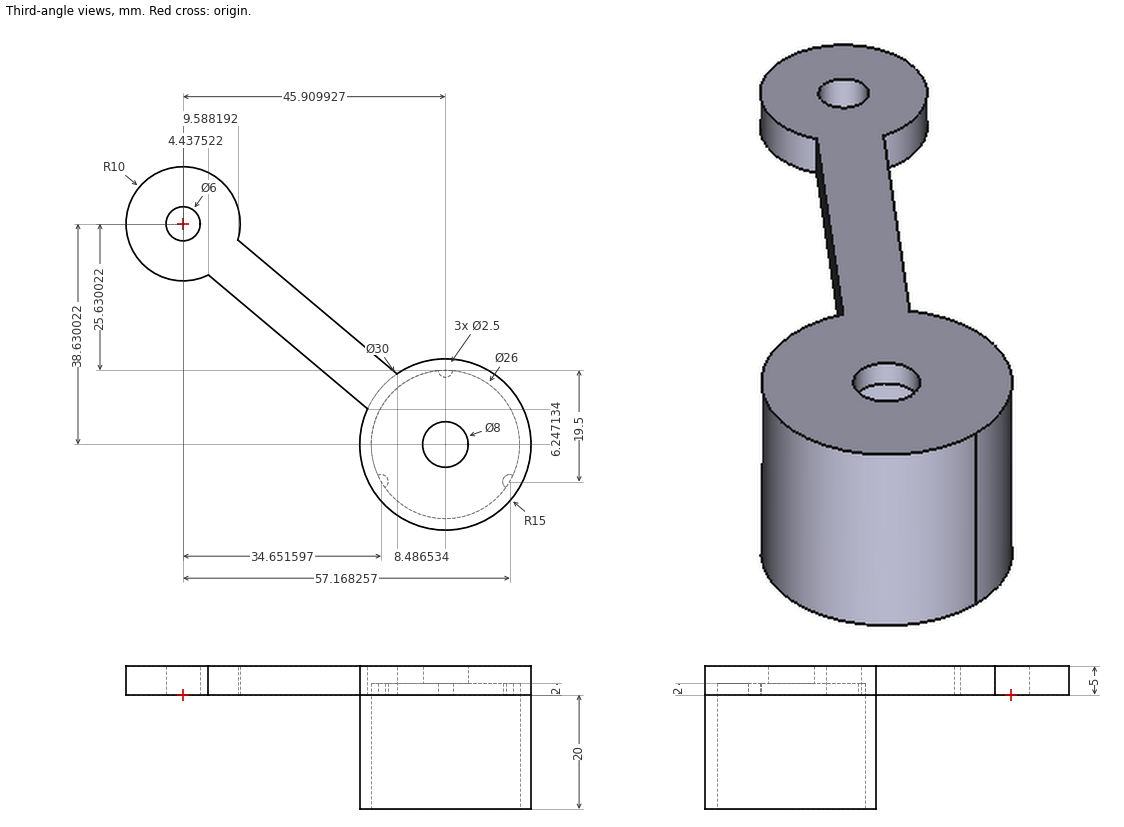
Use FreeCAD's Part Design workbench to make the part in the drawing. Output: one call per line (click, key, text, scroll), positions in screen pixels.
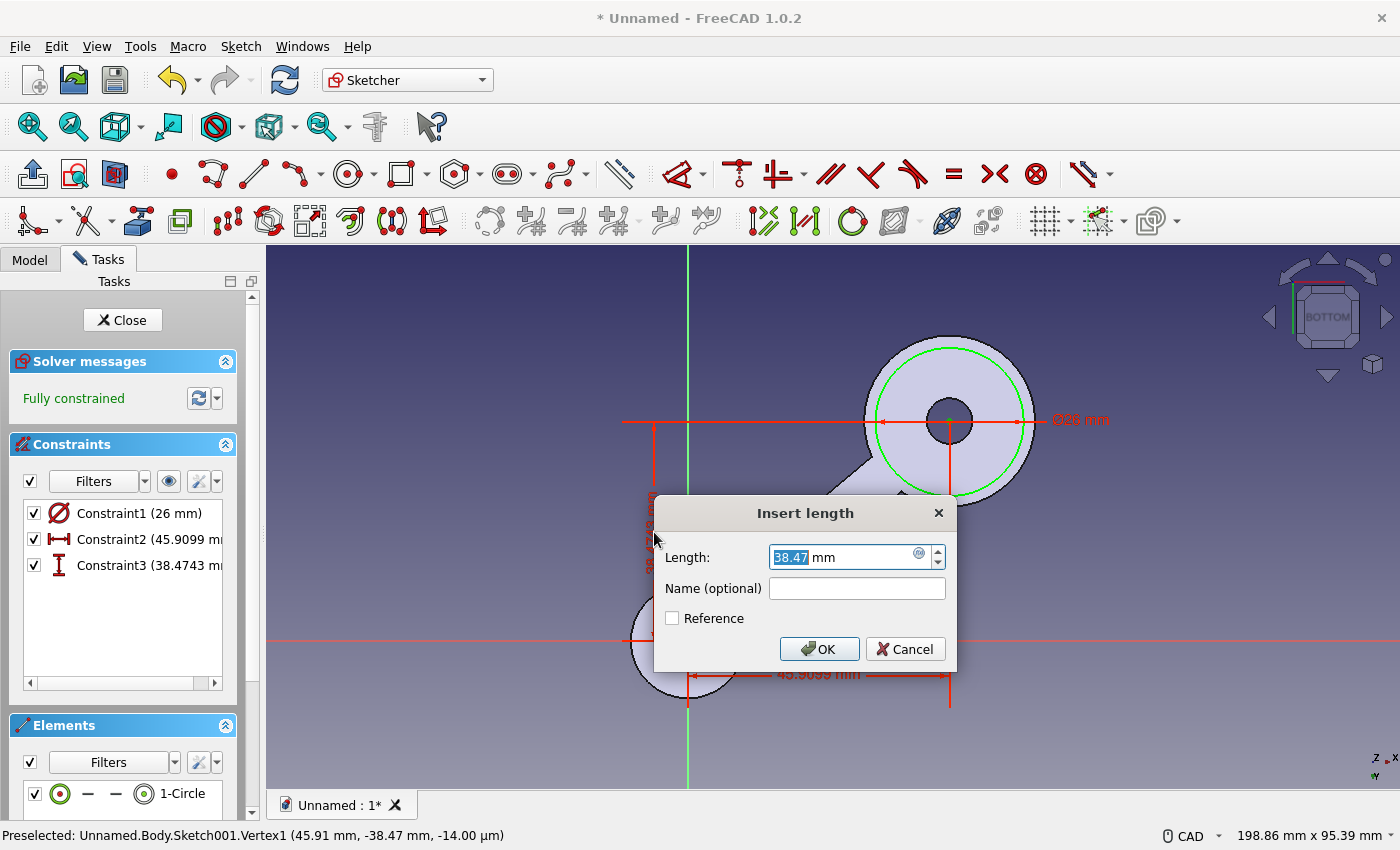
text(38.630022)
key(Return)
key(Escape)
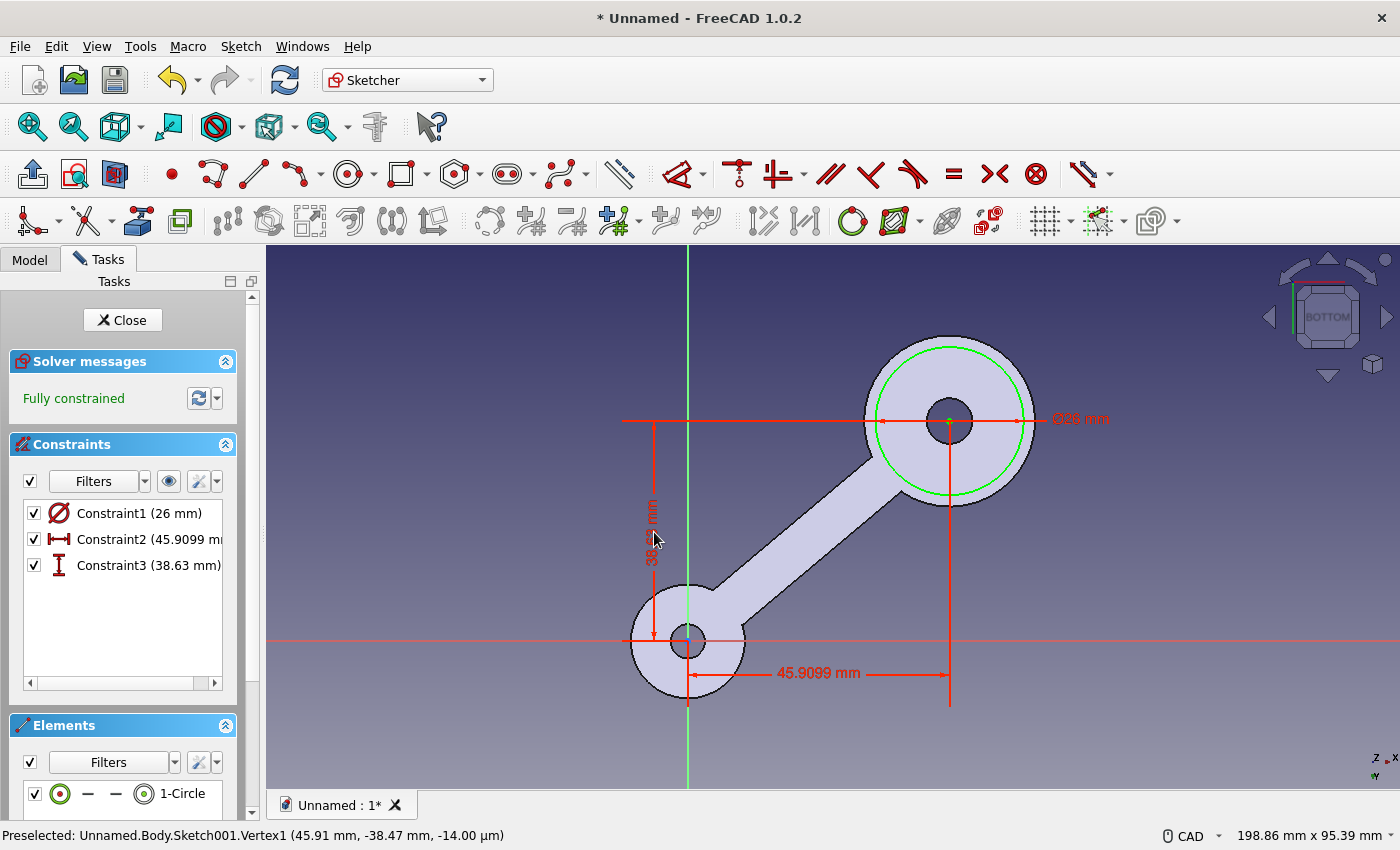
click(123, 320)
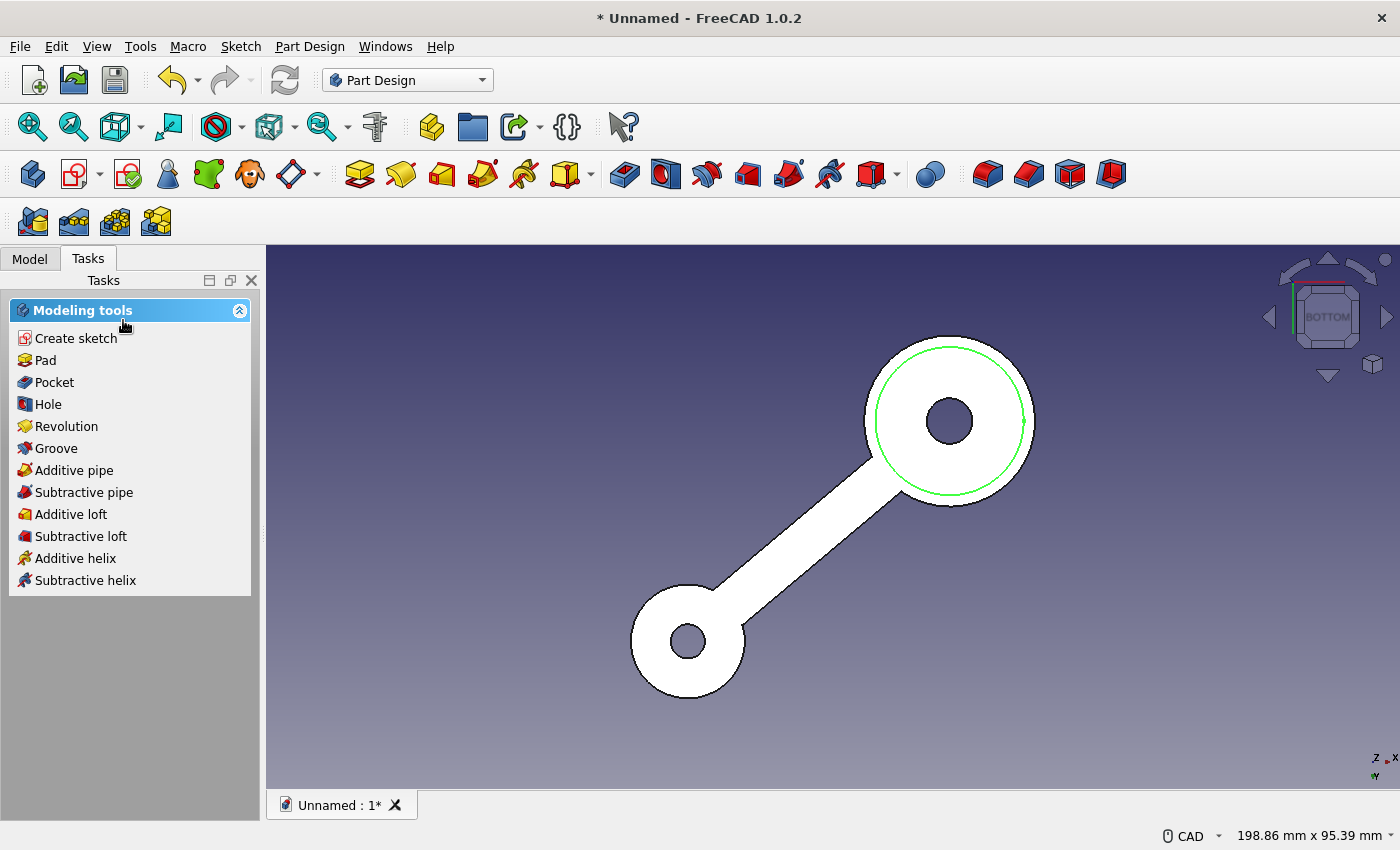
click(625, 174)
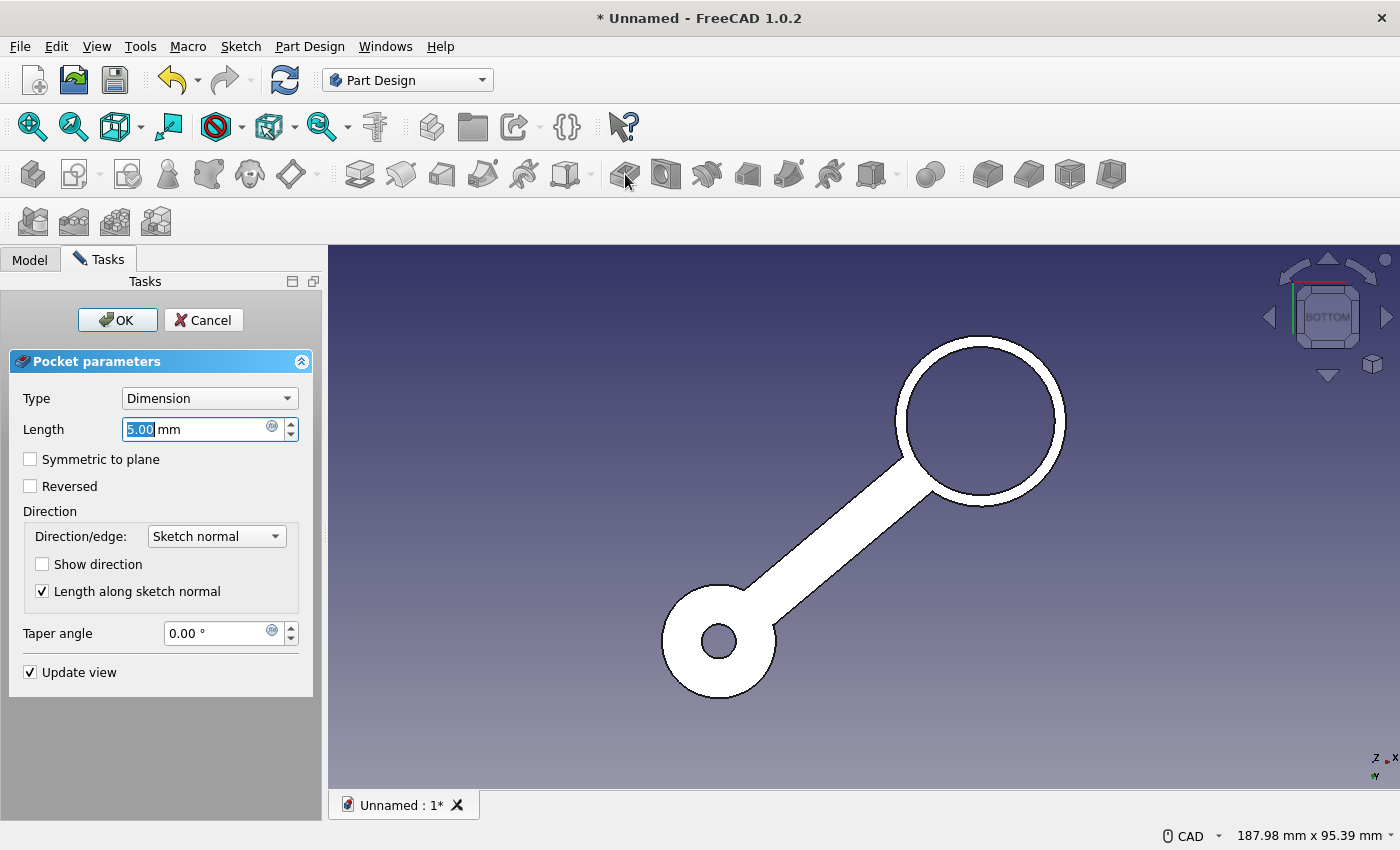
text(2)
key(Tab)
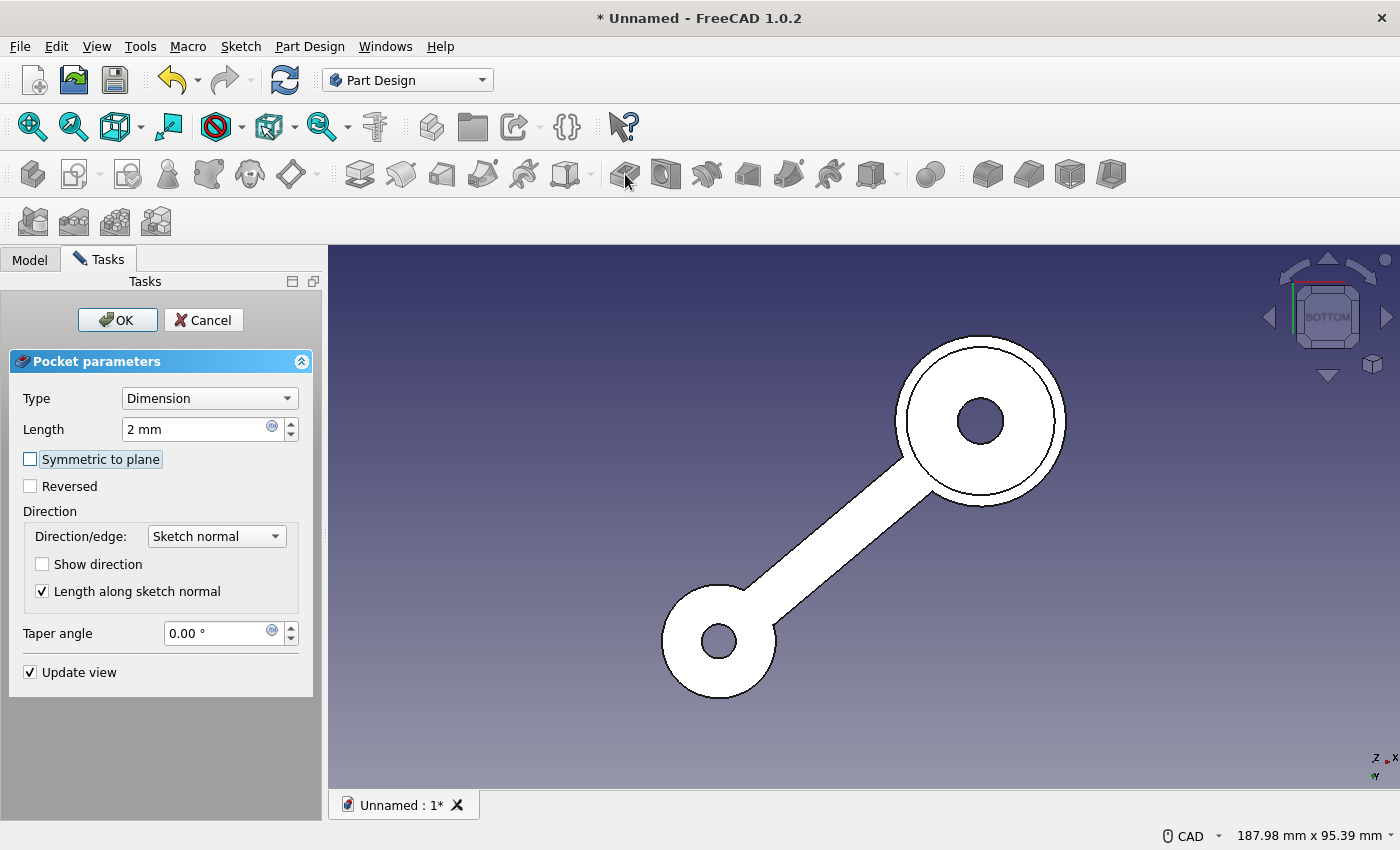
click(118, 320)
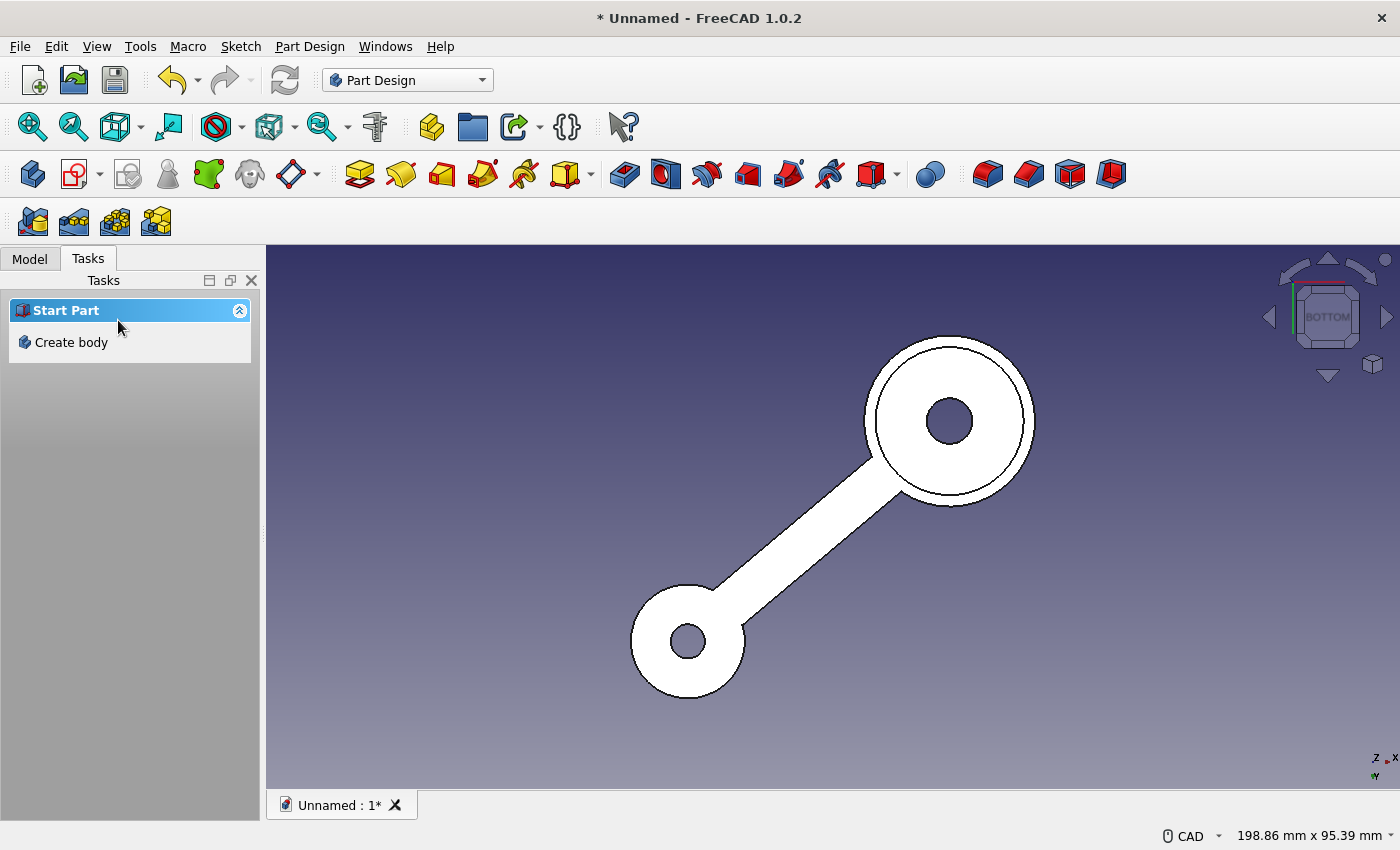
click(775, 568)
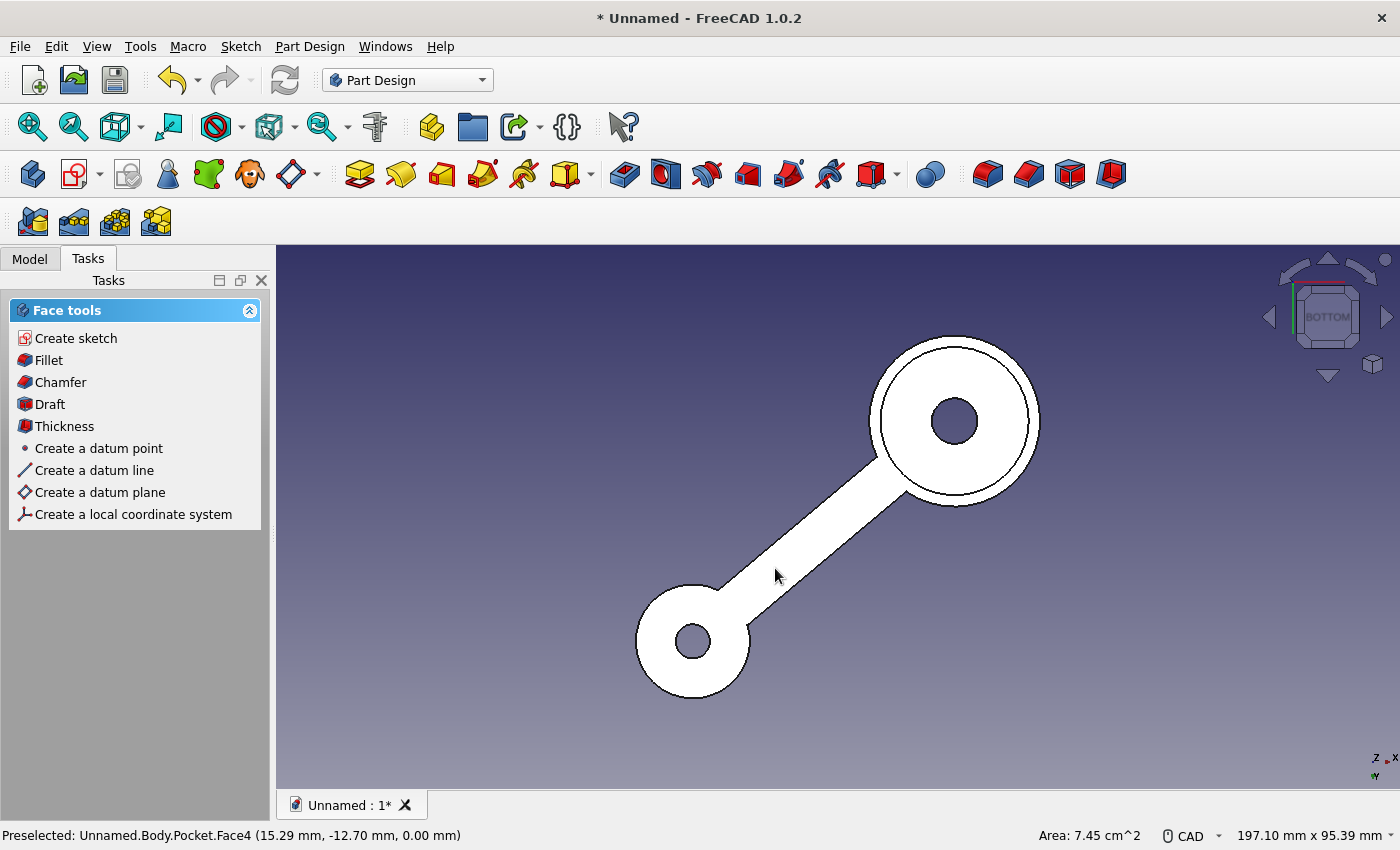
click(74, 174)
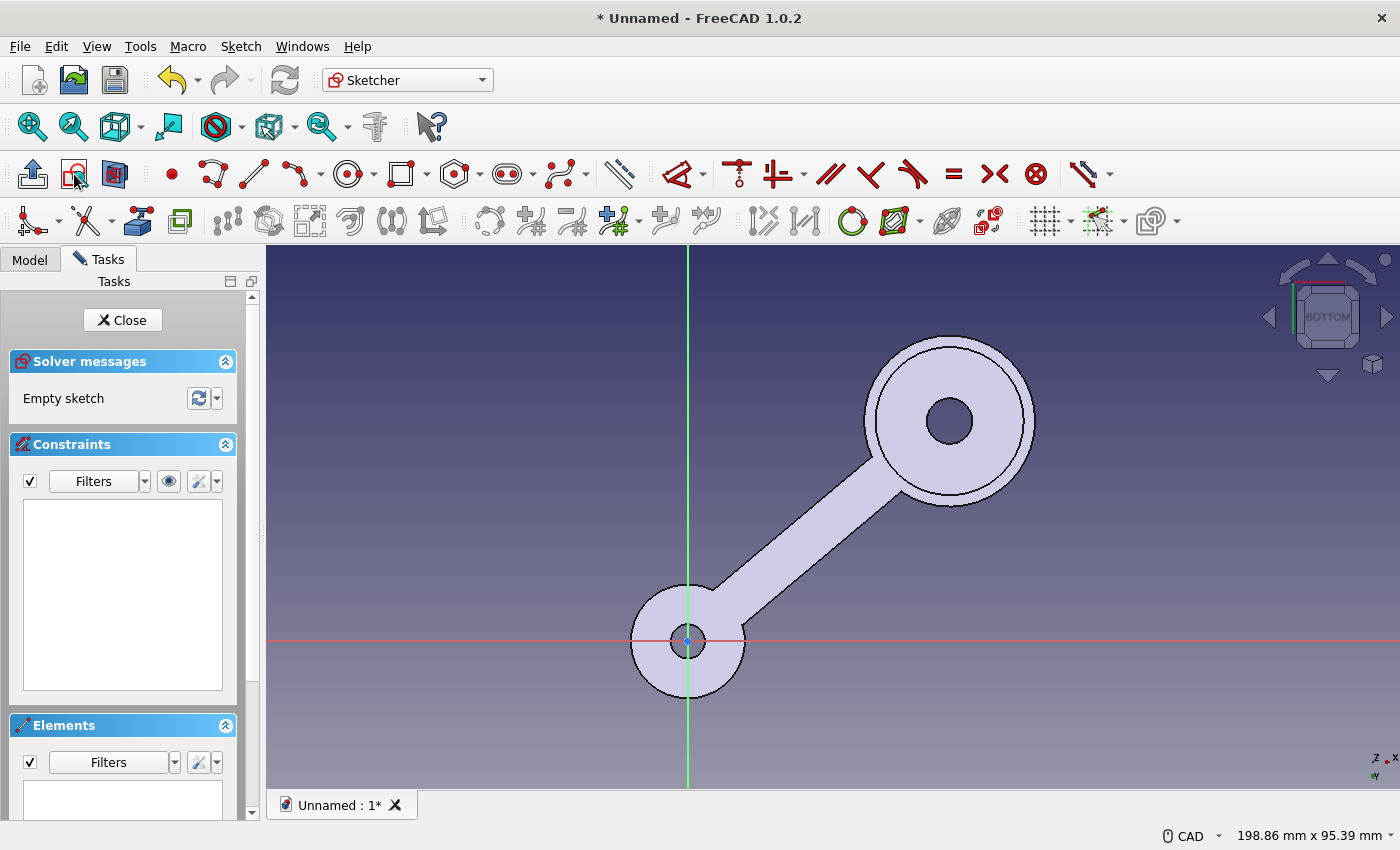
key(g)
key(c)